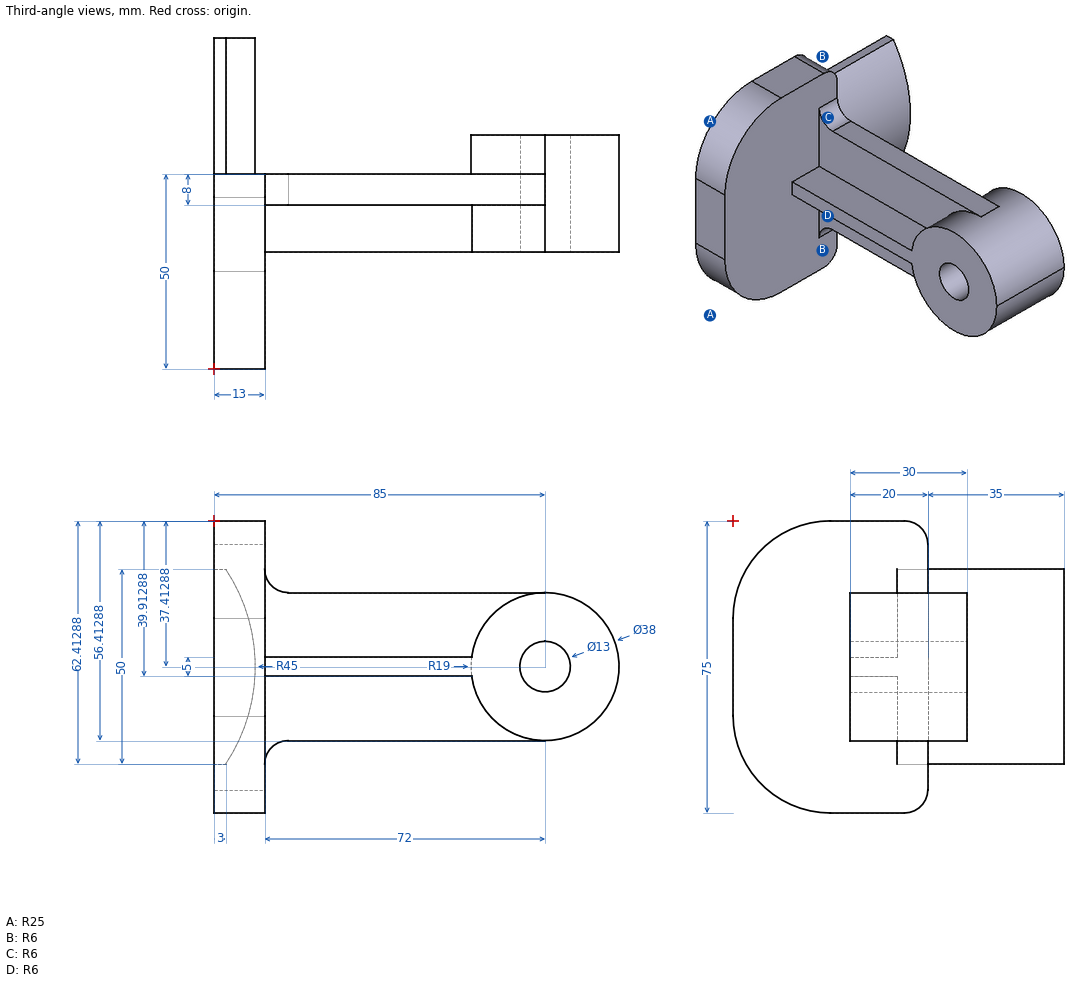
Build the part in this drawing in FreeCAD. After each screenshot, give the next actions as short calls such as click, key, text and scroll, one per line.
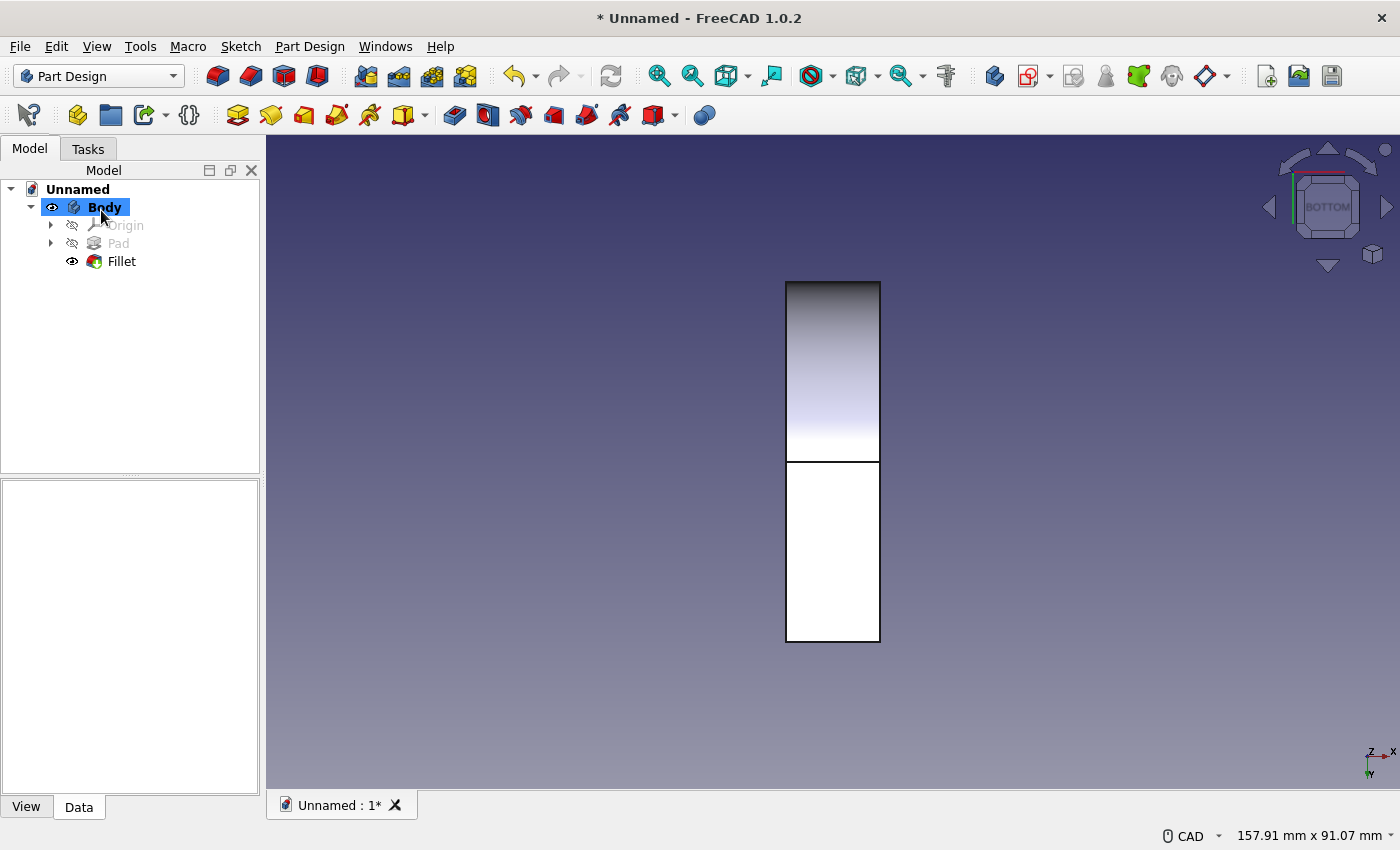
click(833, 641)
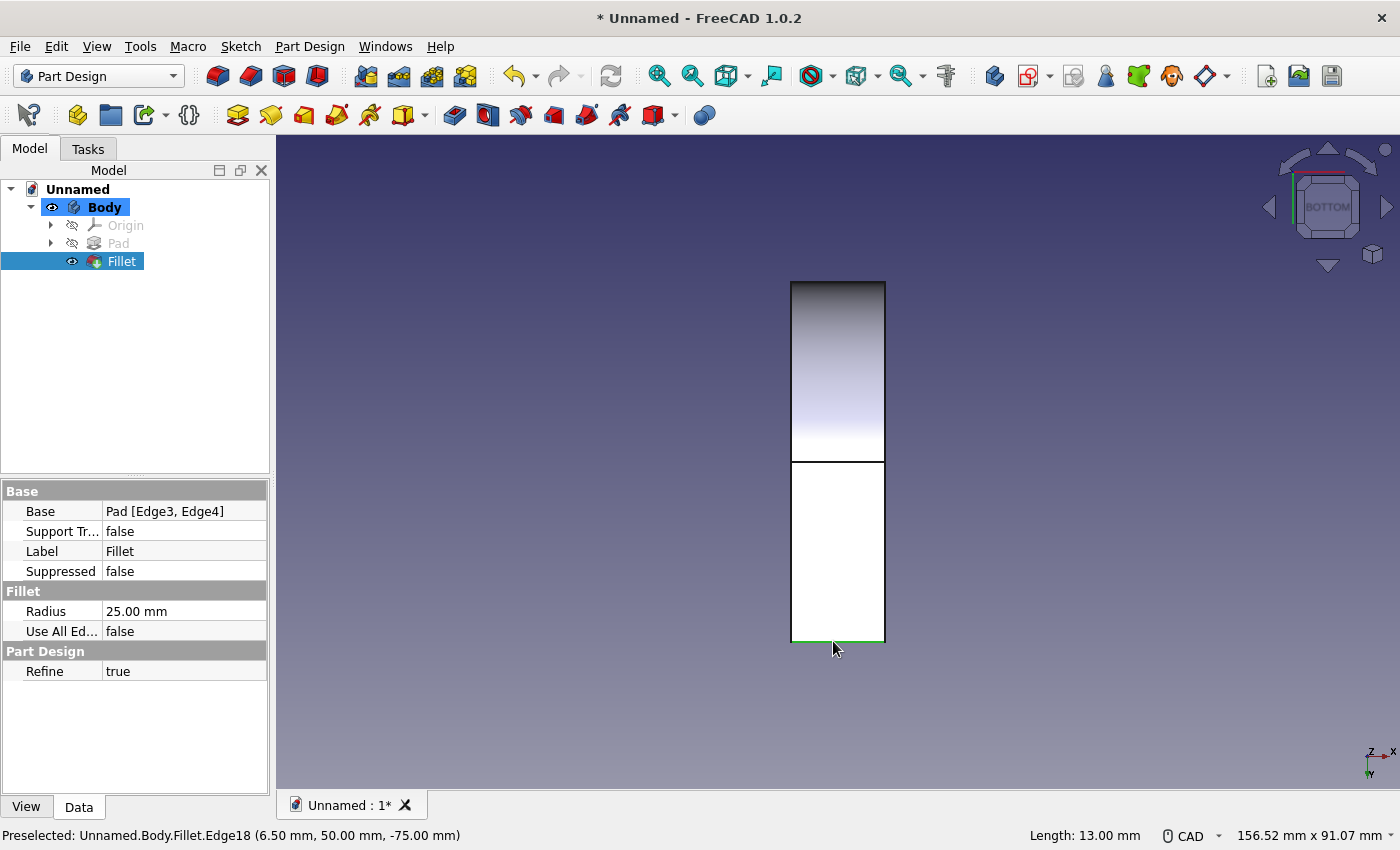
key(4)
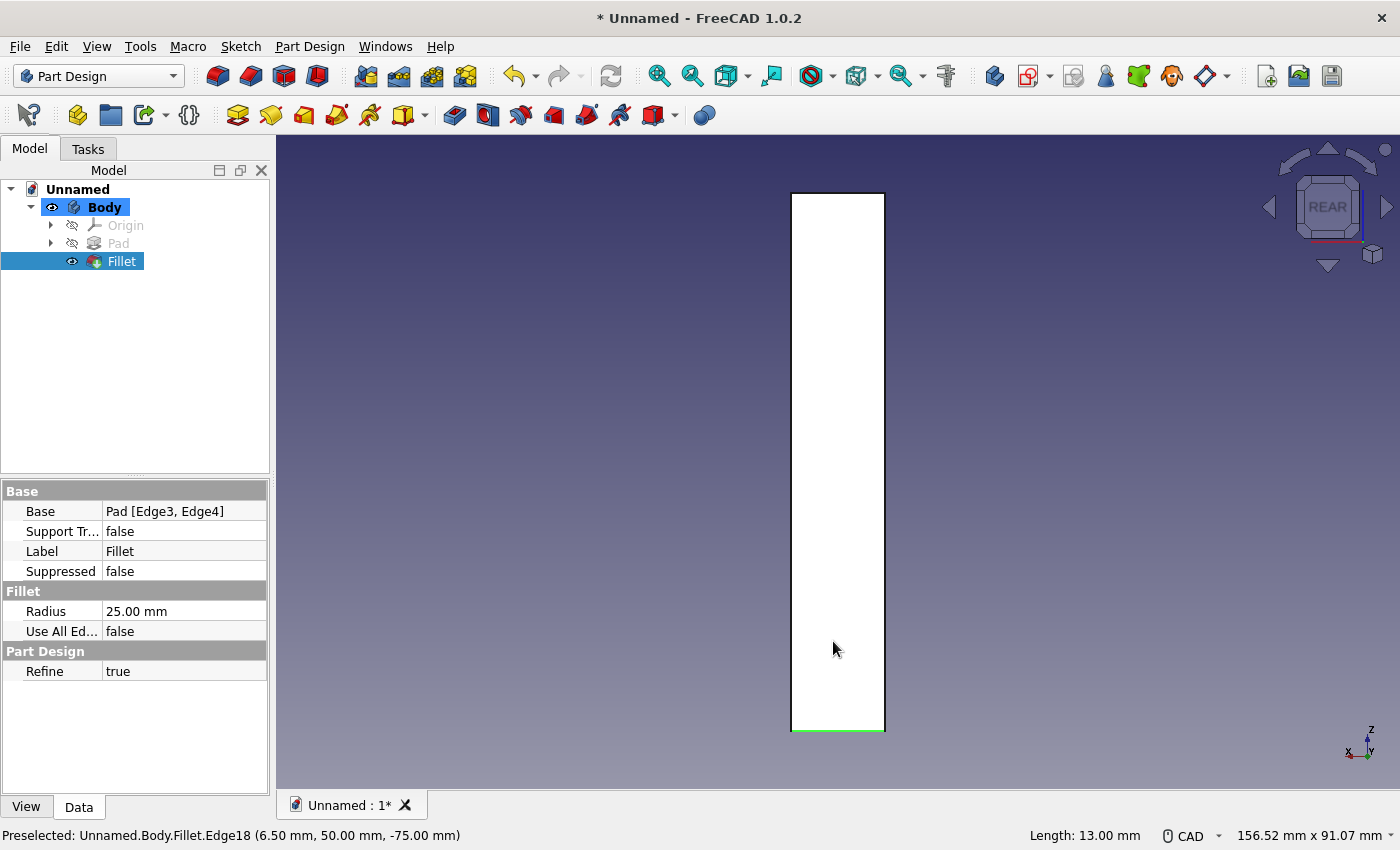
click(838, 192, ctrl)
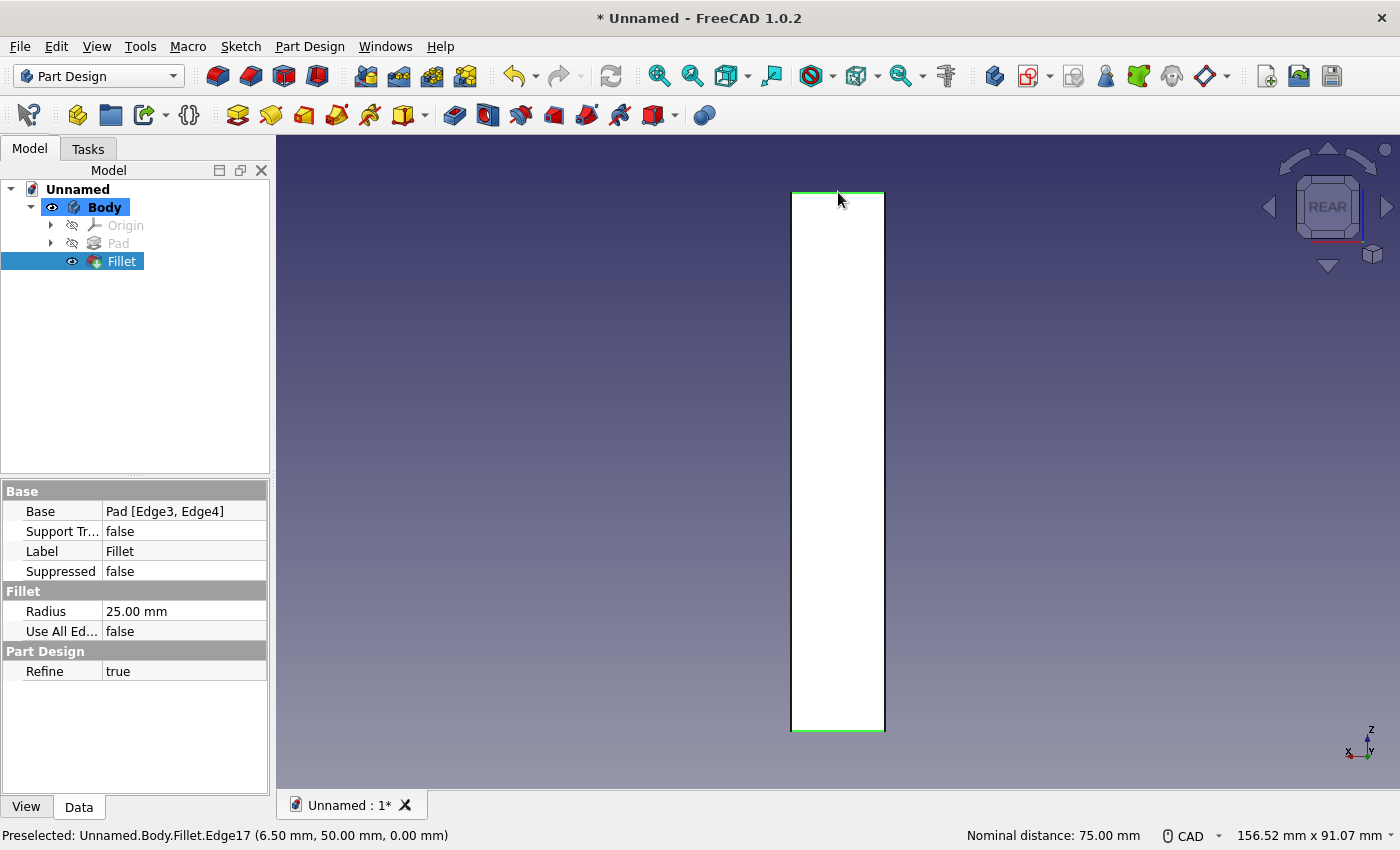
click(218, 76)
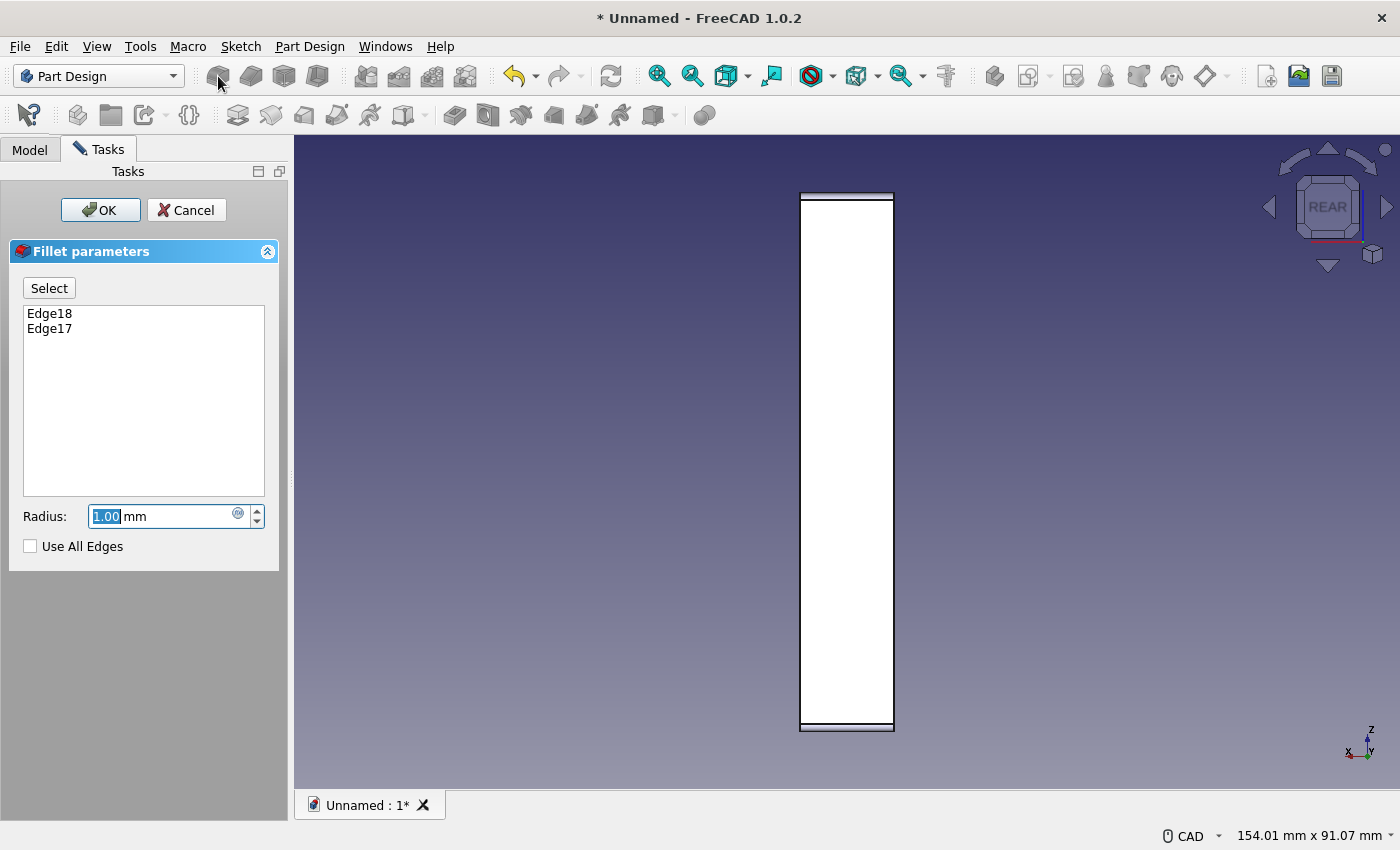
text(6)
key(Tab)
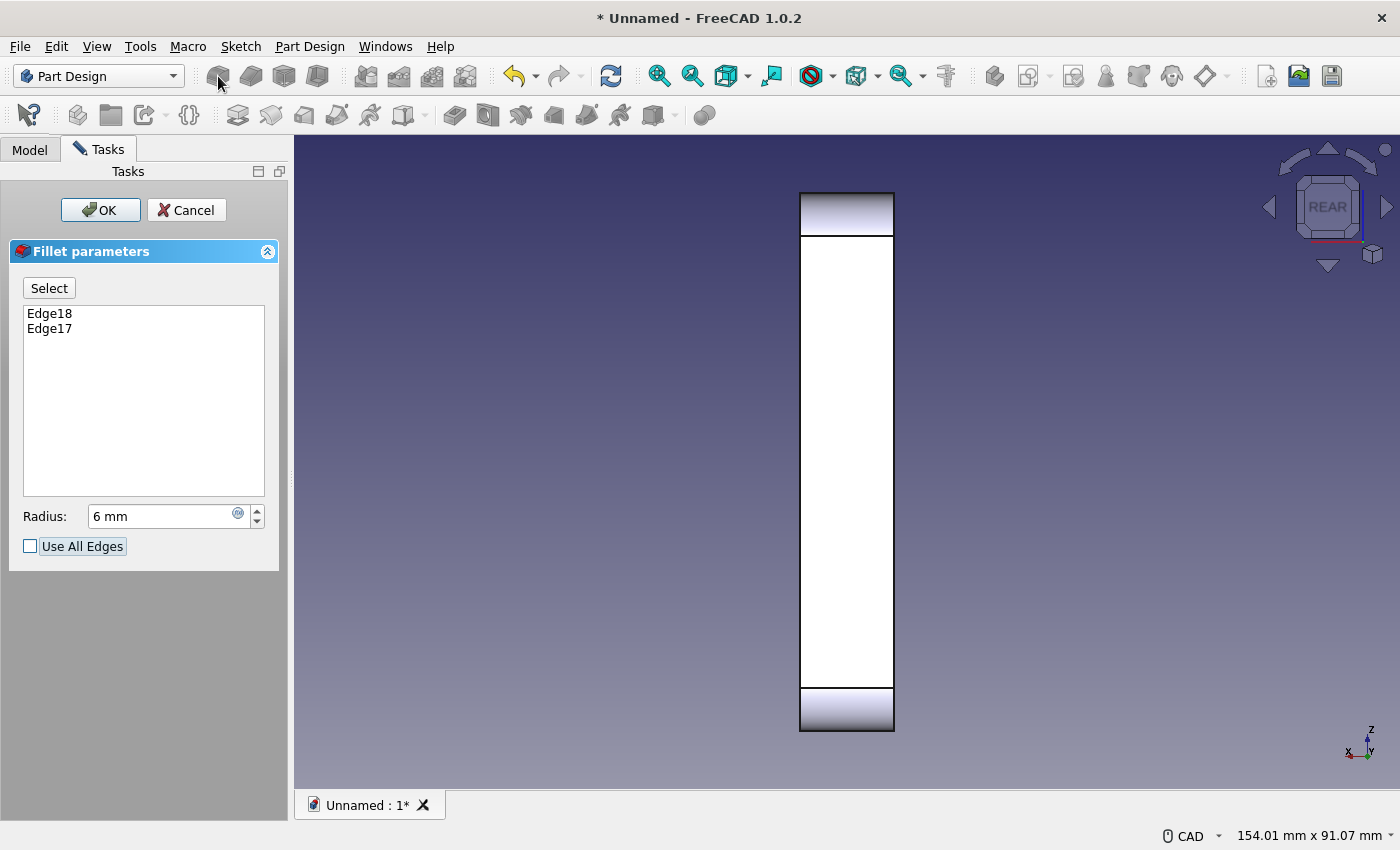
click(101, 210)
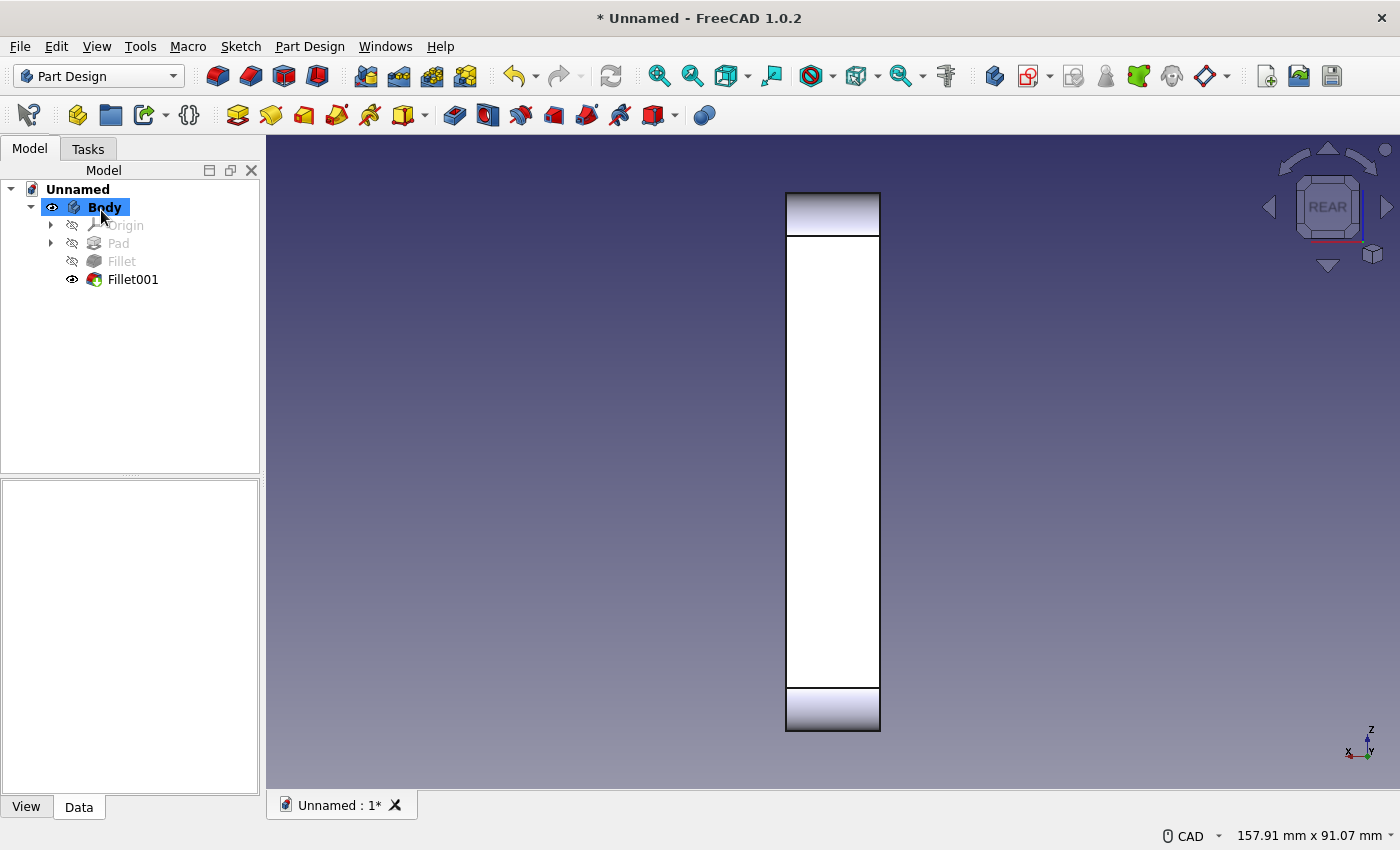
click(833, 332)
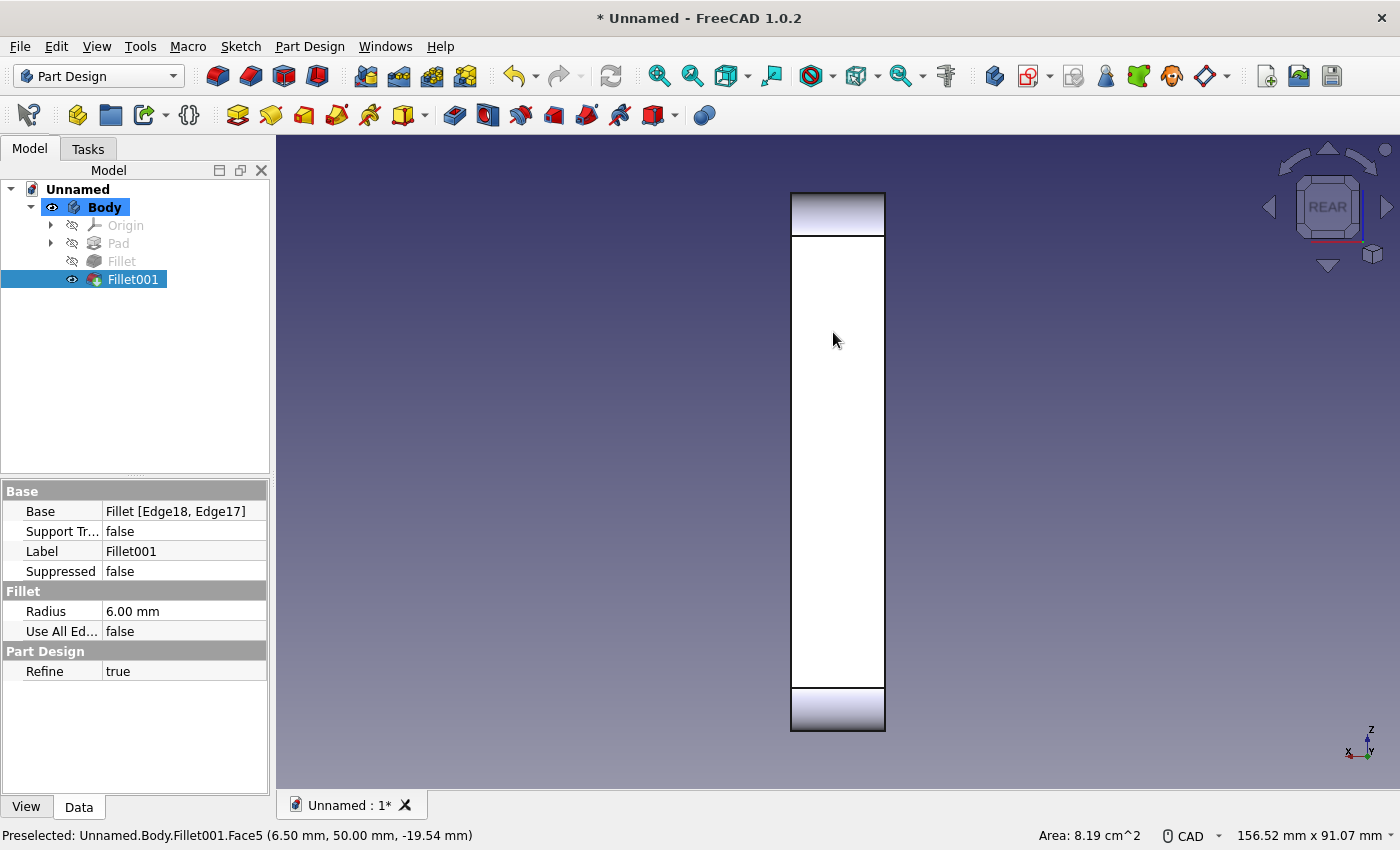
click(1028, 76)